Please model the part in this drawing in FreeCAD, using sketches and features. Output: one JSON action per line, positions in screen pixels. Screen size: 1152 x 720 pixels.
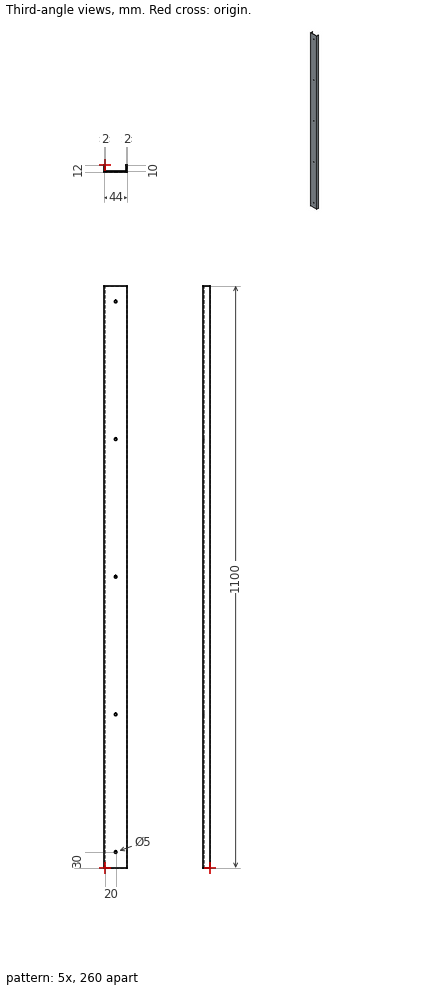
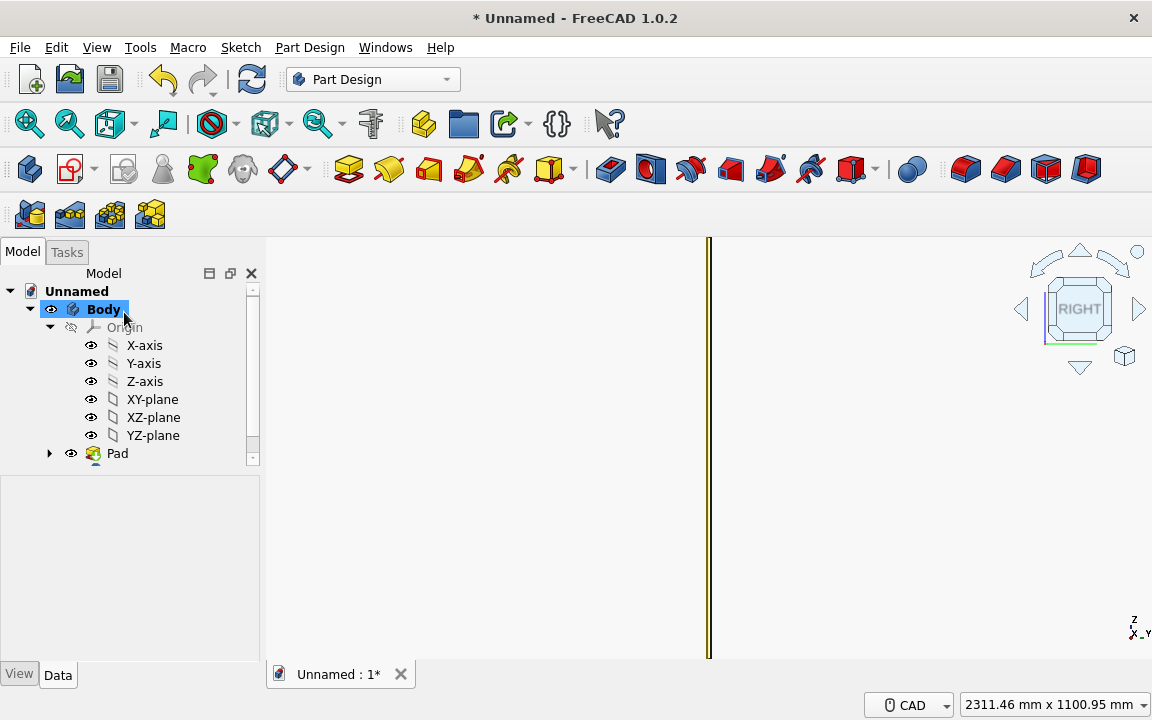
{"action": "scroll", "coordinate": [100, 377], "scroll_direction": "down", "scroll_amount": 3}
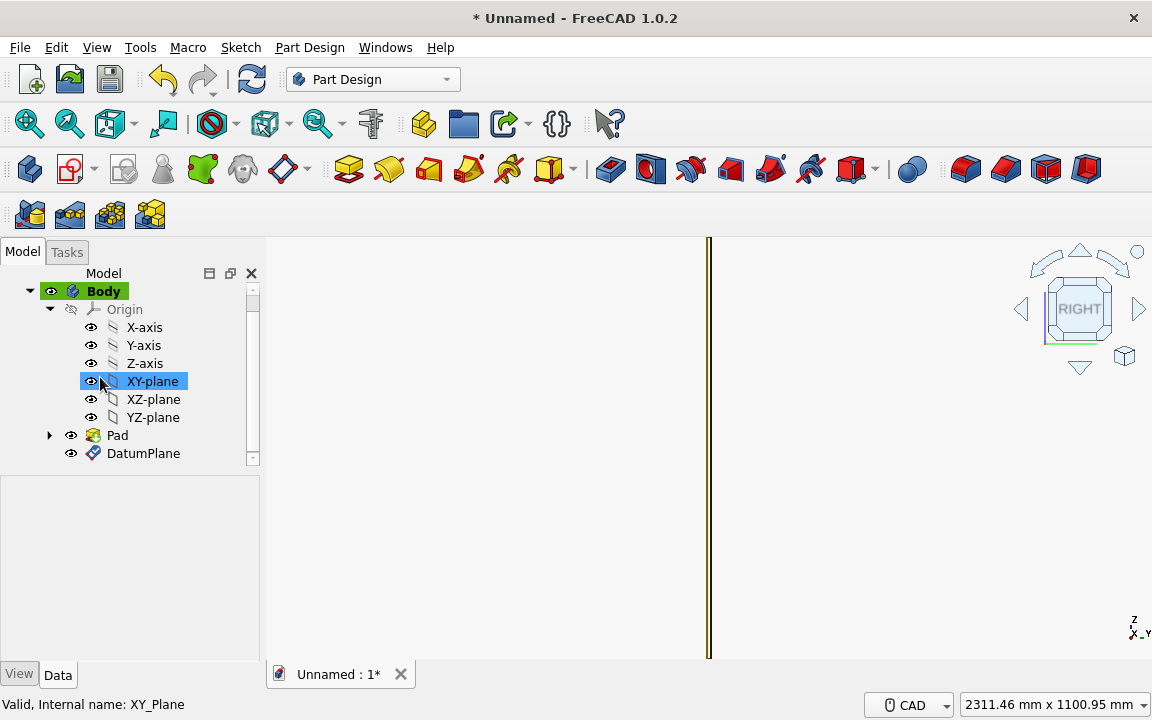
{"action": "left_click", "coordinate": [116, 453]}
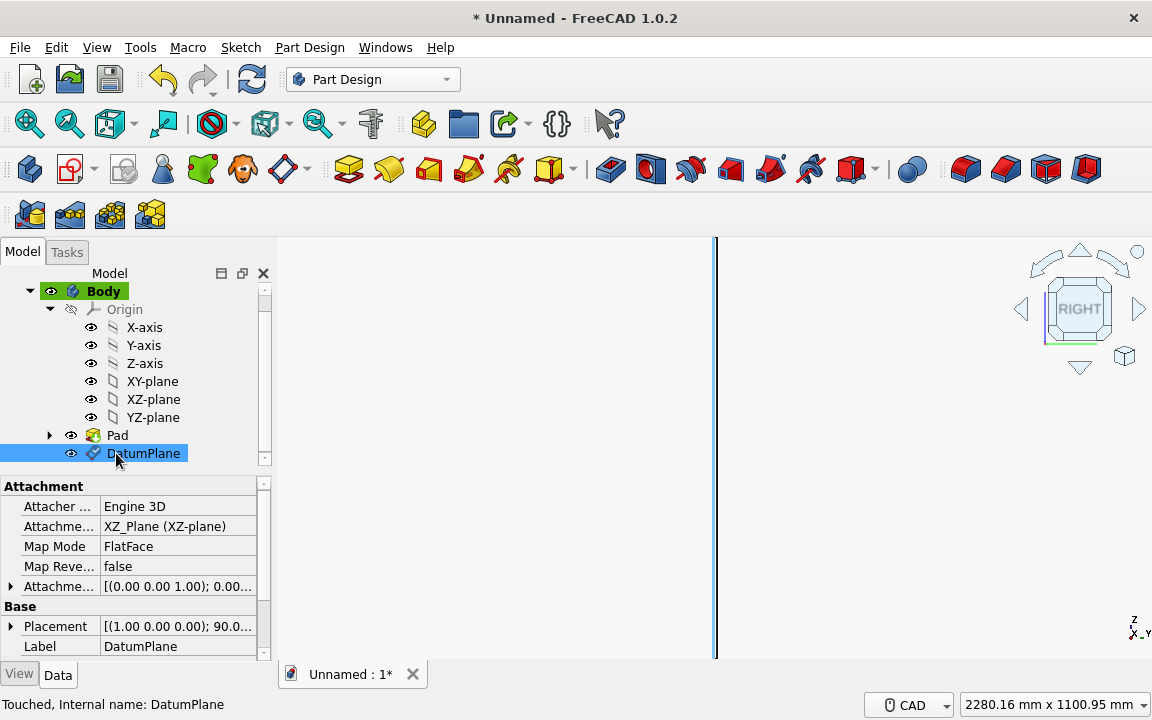
{"action": "left_click", "coordinate": [70, 170]}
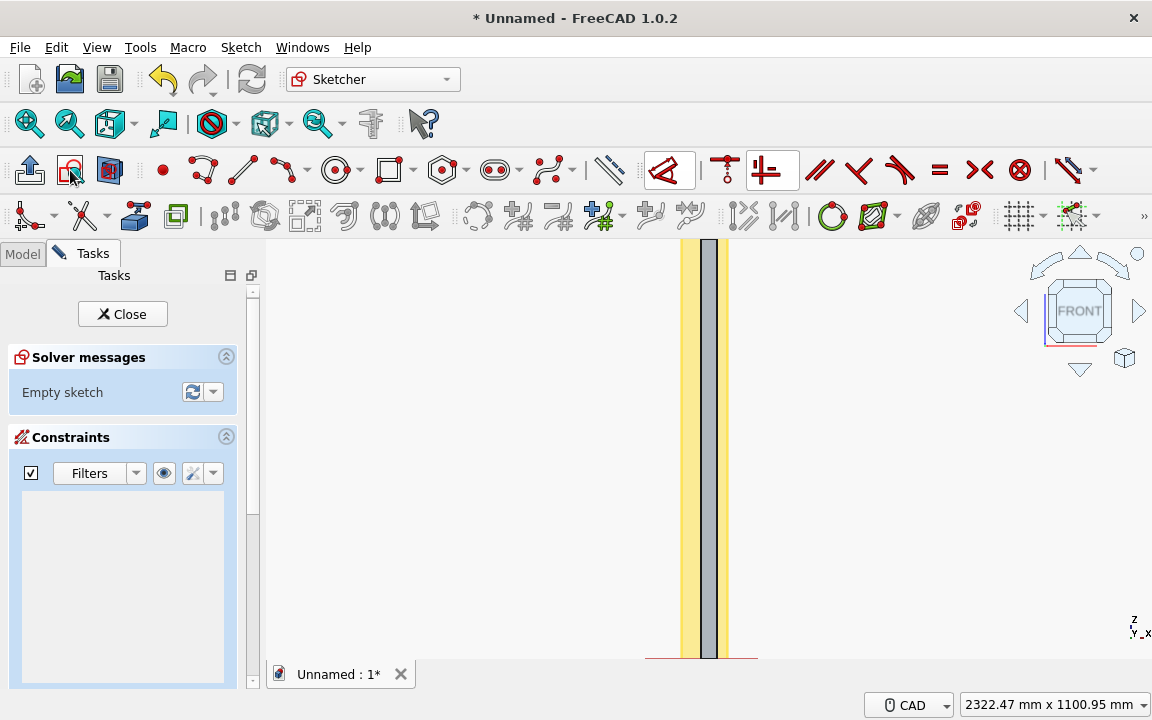
{"action": "left_click", "coordinate": [110, 170]}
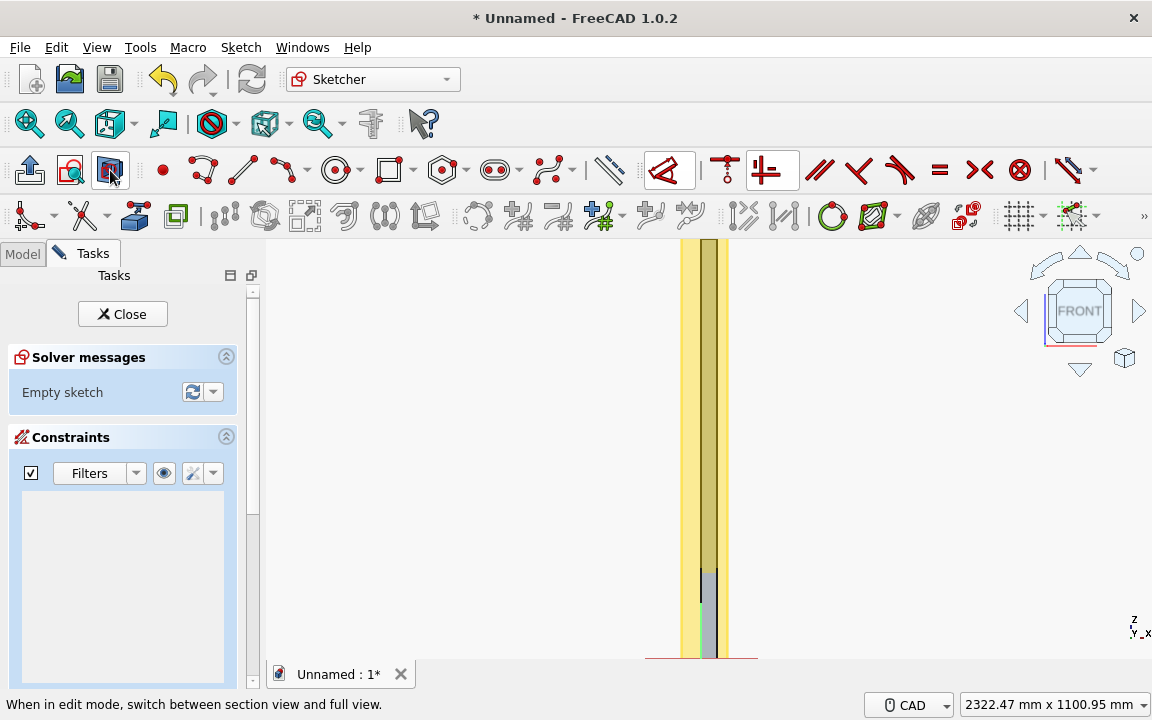
{"action": "scroll", "coordinate": [640, 449], "scroll_direction": "down", "scroll_amount": 5}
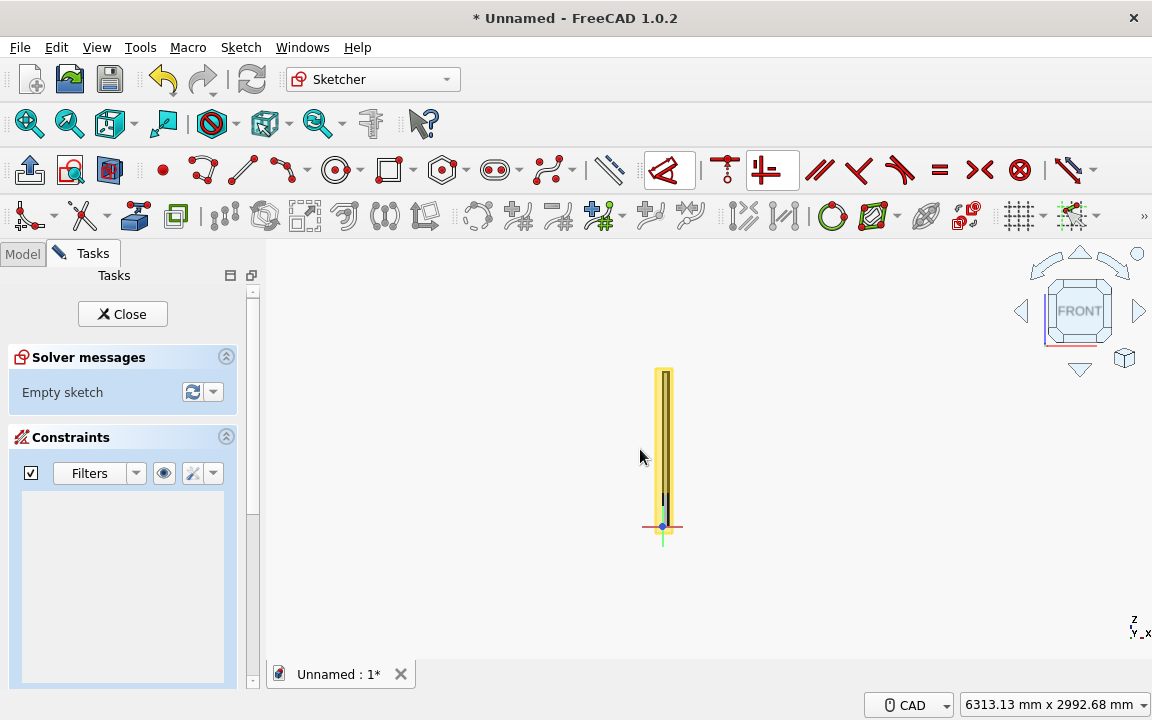
{"action": "scroll", "coordinate": [667, 526], "scroll_direction": "up", "scroll_amount": 15}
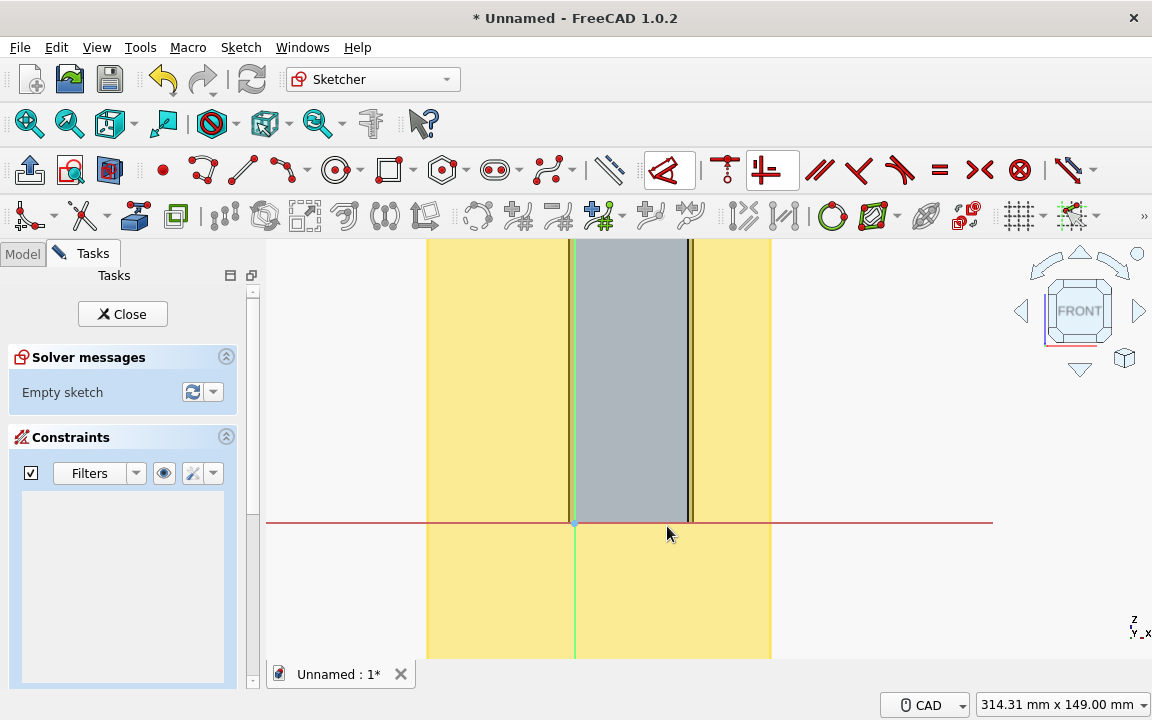
{"action": "scroll", "coordinate": [631, 438], "scroll_direction": "up", "scroll_amount": 15}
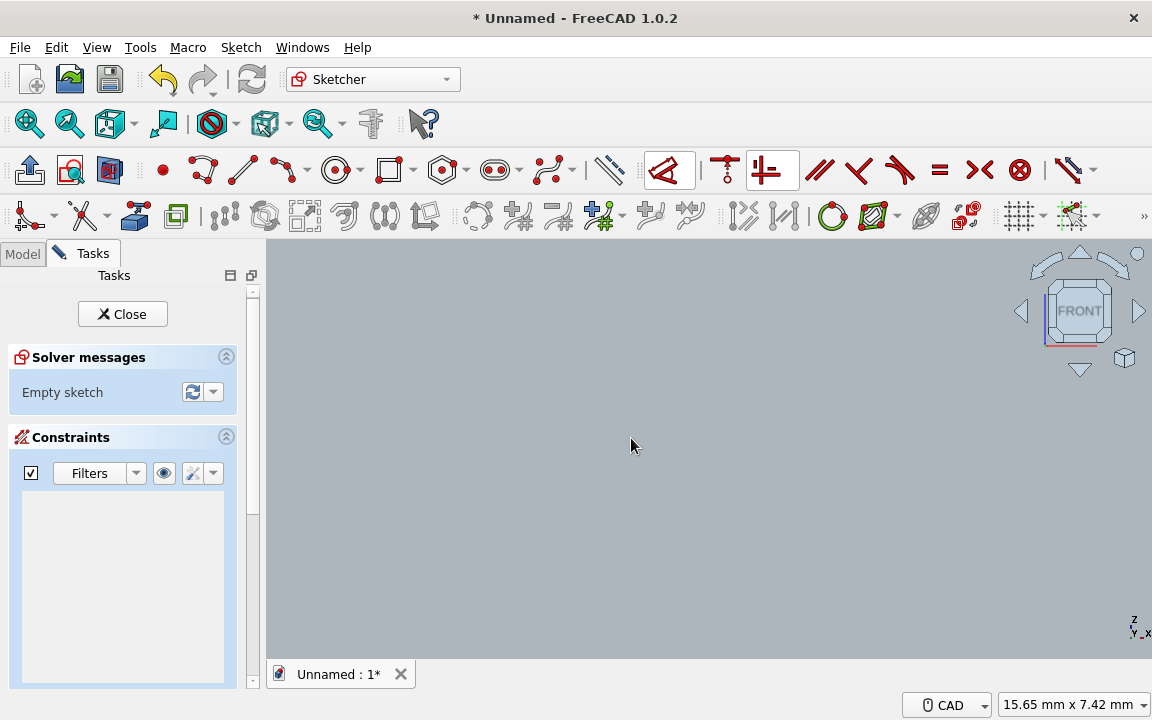
{"action": "left_click", "coordinate": [336, 170]}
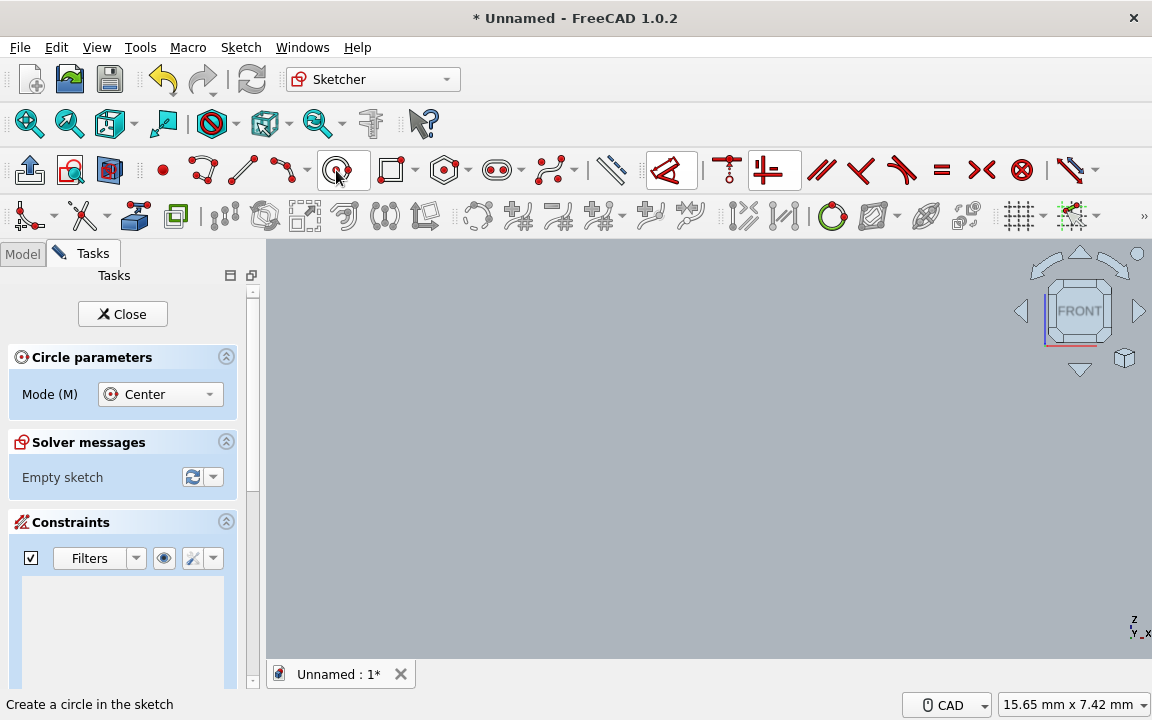
{"action": "left_click", "coordinate": [628, 439]}
{"action": "left_click", "coordinate": [728, 339]}
{"action": "key", "text": "Escape"}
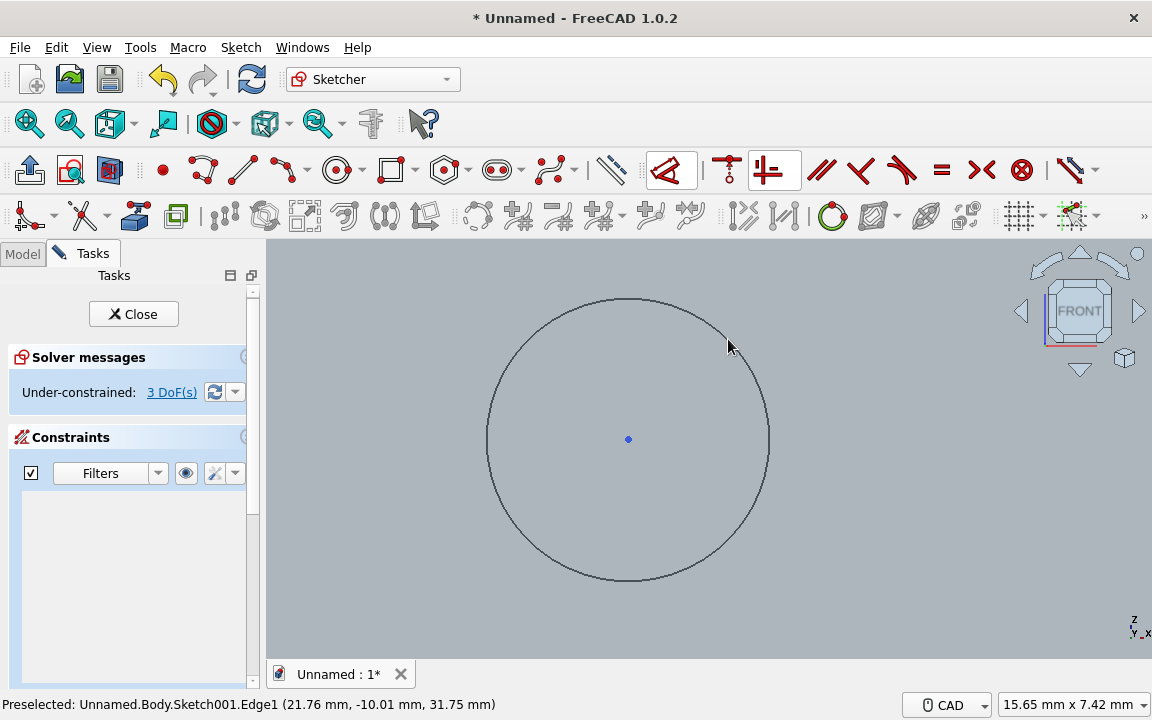
{"action": "left_click", "coordinate": [728, 340]}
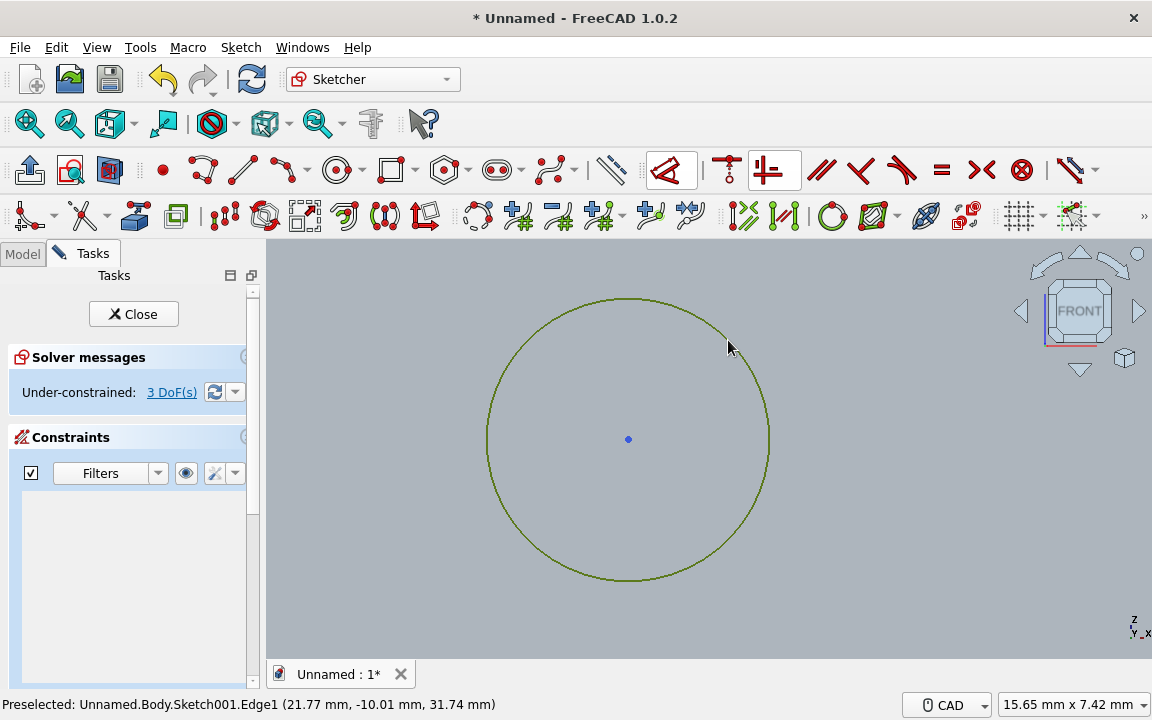
{"action": "key", "text": "k o"}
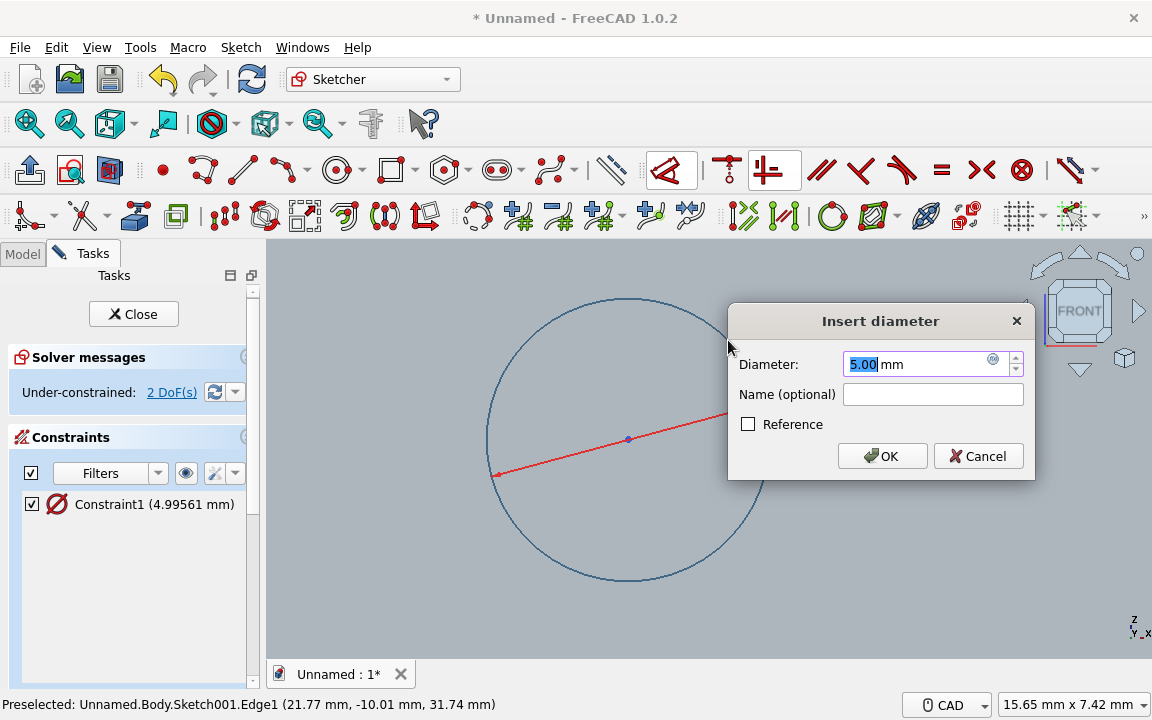
{"action": "type", "text": "5"}
{"action": "key", "text": "Return"}